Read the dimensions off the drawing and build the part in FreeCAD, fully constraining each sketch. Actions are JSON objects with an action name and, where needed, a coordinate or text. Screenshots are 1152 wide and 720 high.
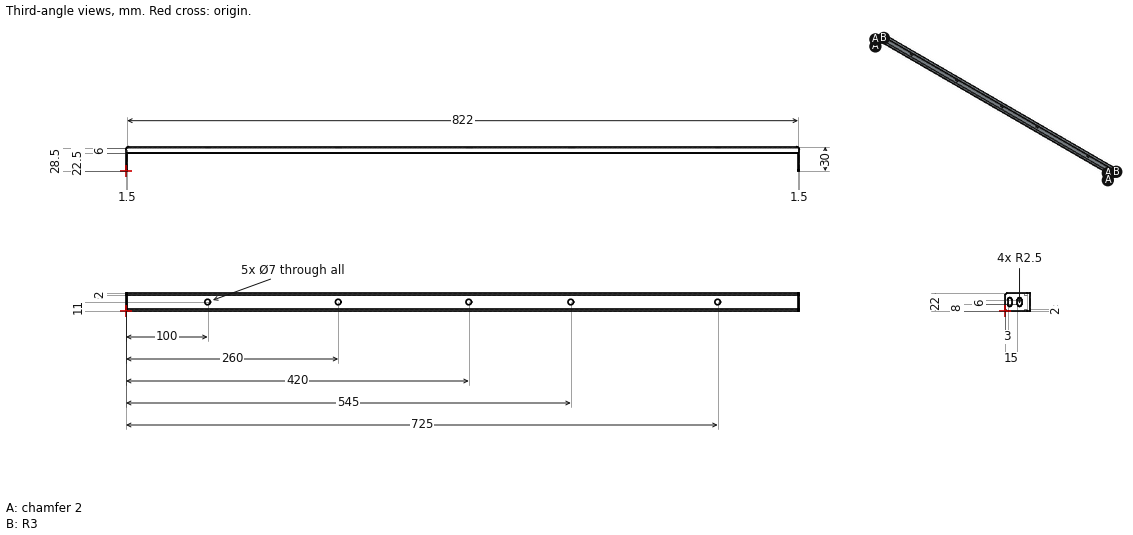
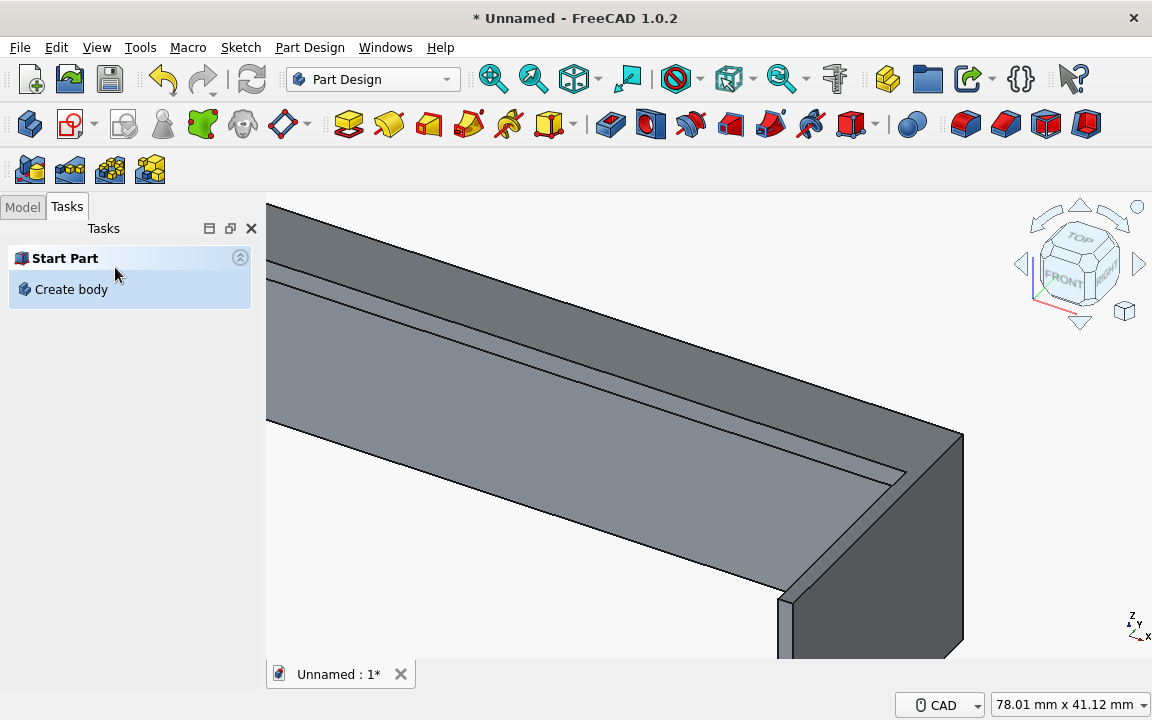
{"action": "left_click", "coordinate": [494, 80]}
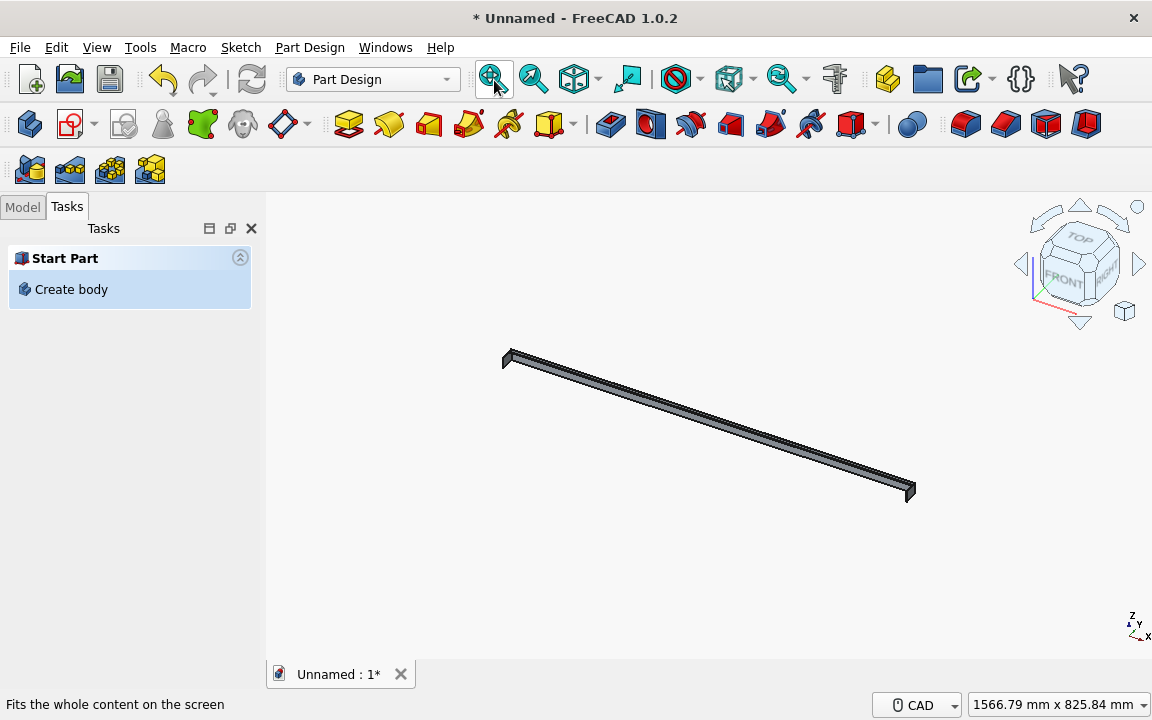
{"action": "key", "text": "5"}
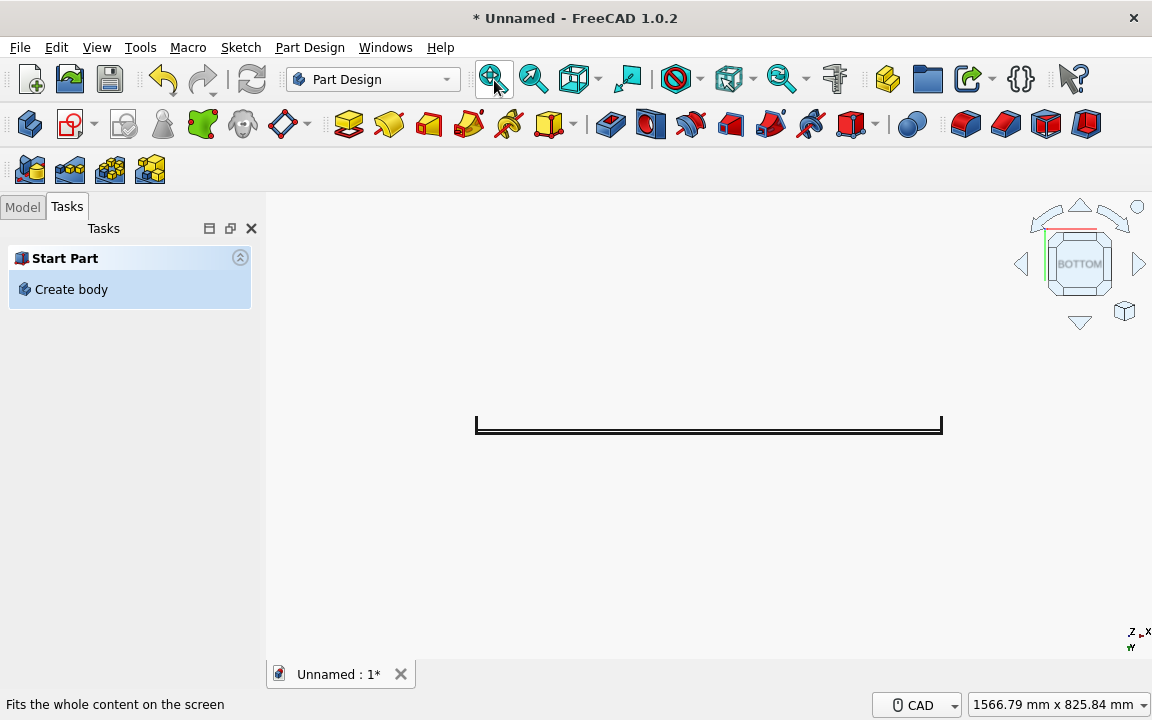
{"action": "scroll", "coordinate": [942, 427], "scroll_direction": "up", "scroll_amount": 15}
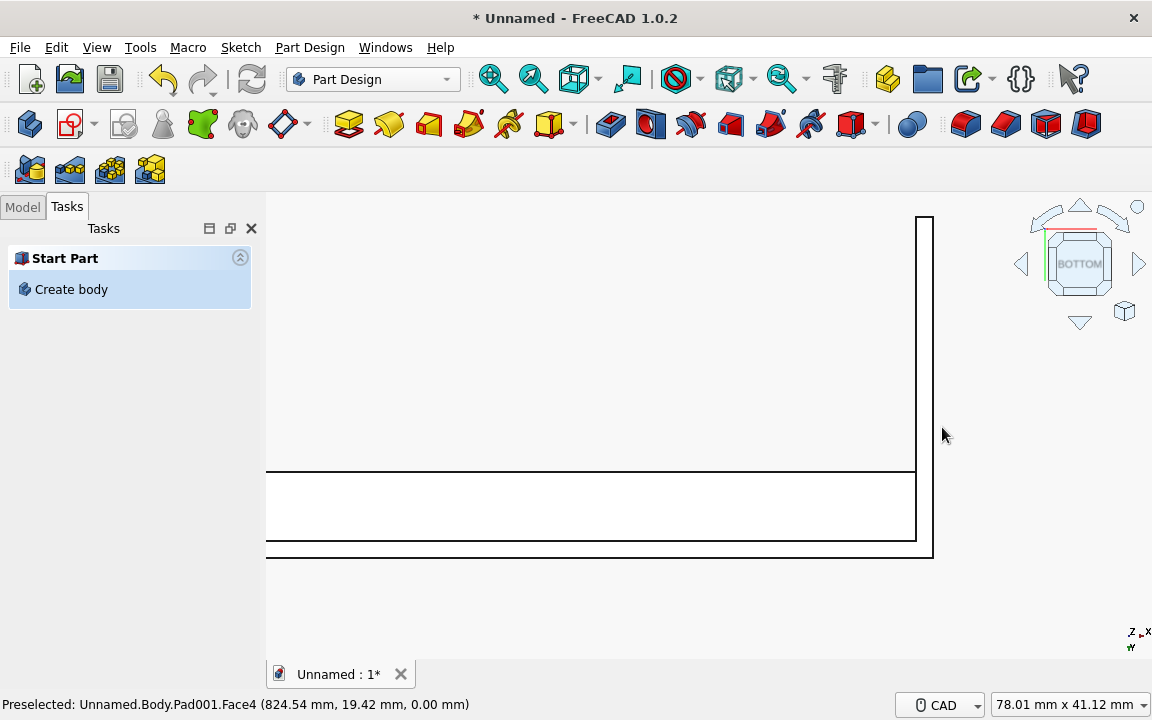
{"action": "scroll", "coordinate": [927, 437], "scroll_direction": "up", "scroll_amount": 4}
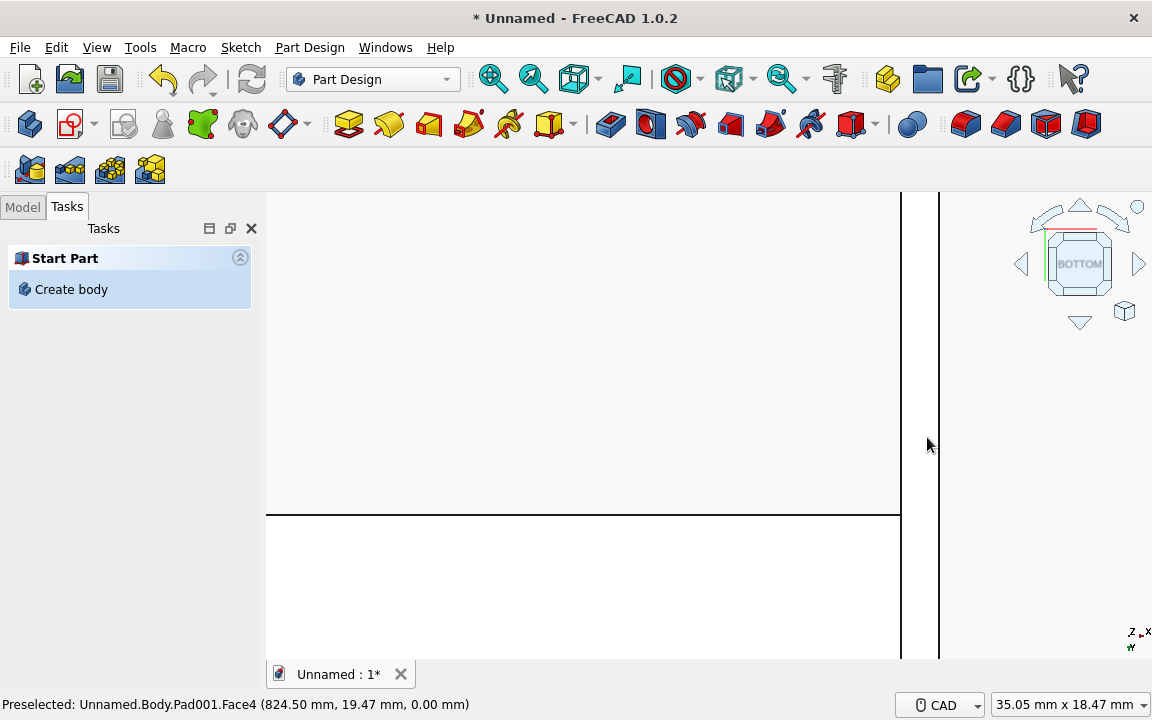
{"action": "left_click", "coordinate": [926, 438]}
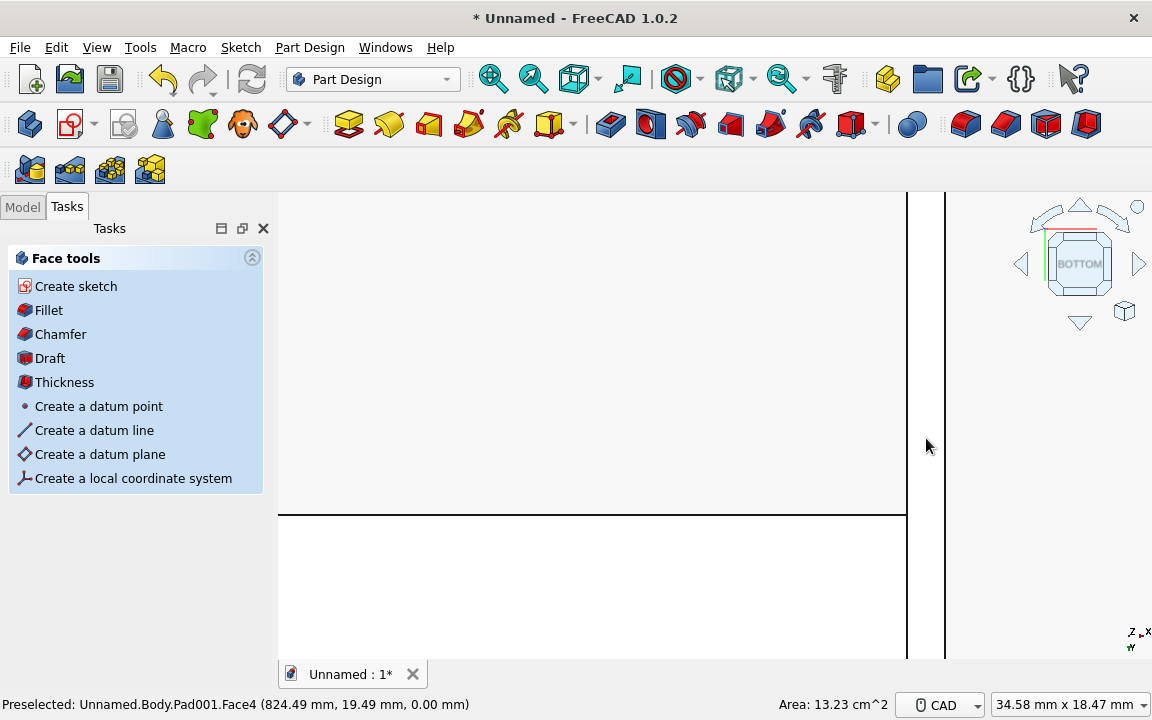
{"action": "left_click", "coordinate": [70, 124]}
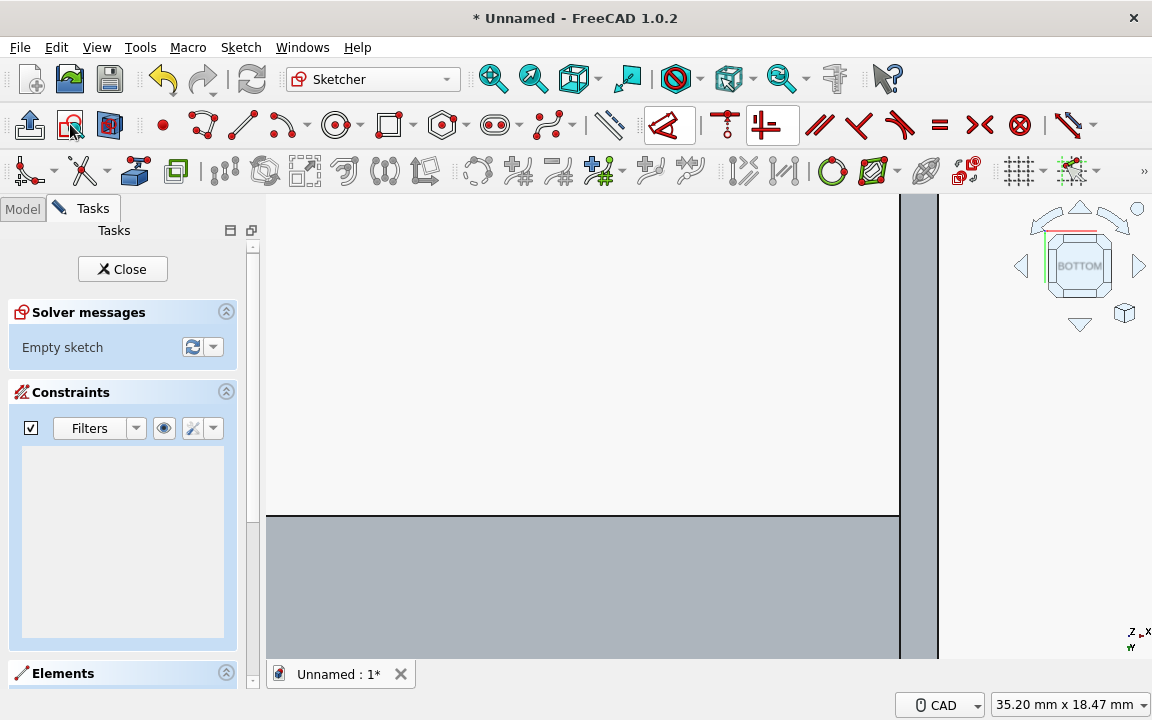
{"action": "scroll", "coordinate": [924, 430], "scroll_direction": "down", "scroll_amount": 18}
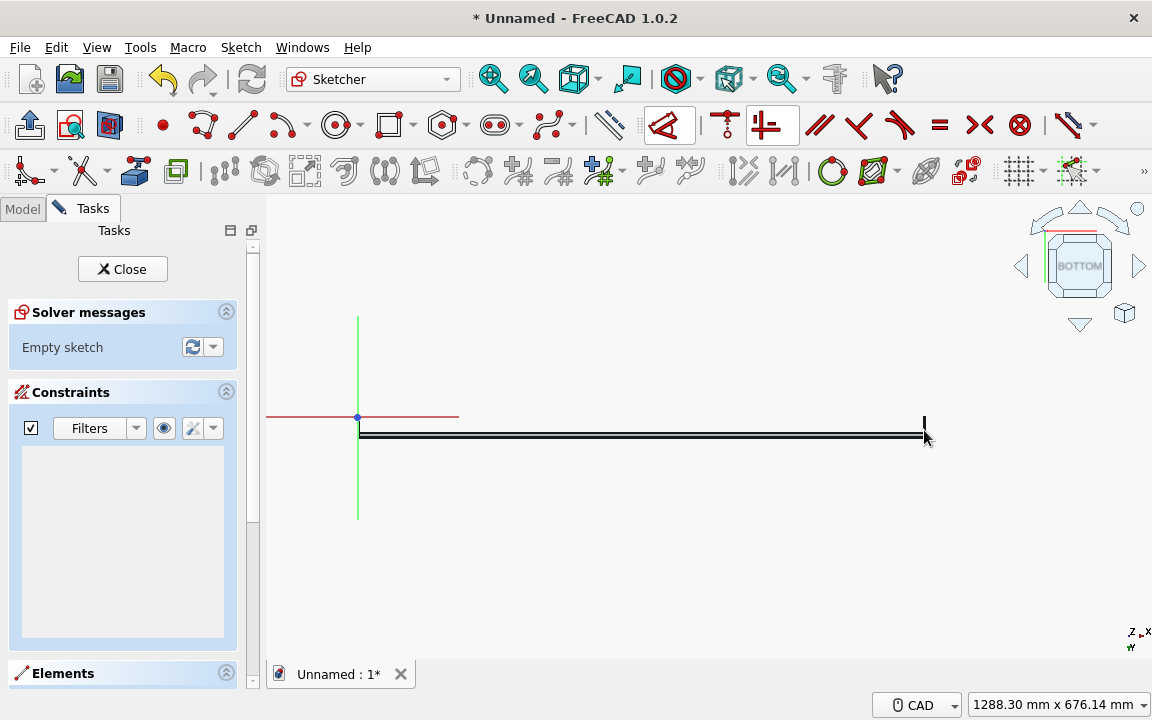
{"action": "left_click", "coordinate": [390, 126]}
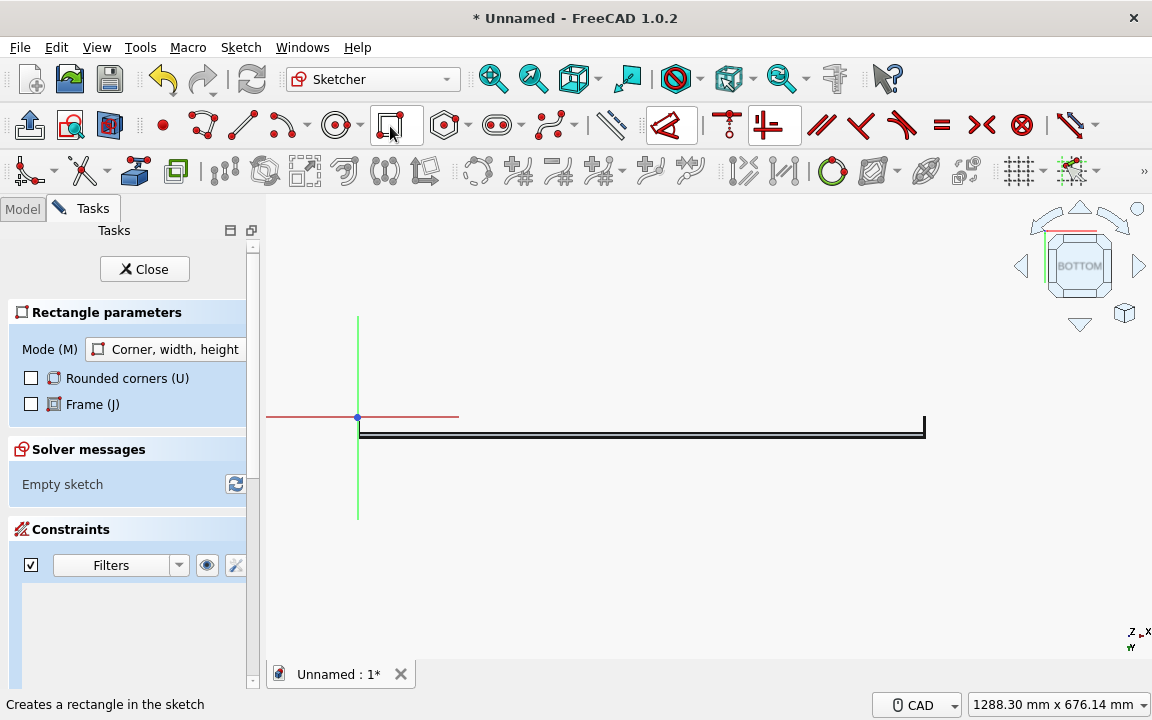
{"action": "scroll", "coordinate": [359, 433], "scroll_direction": "up", "scroll_amount": 14}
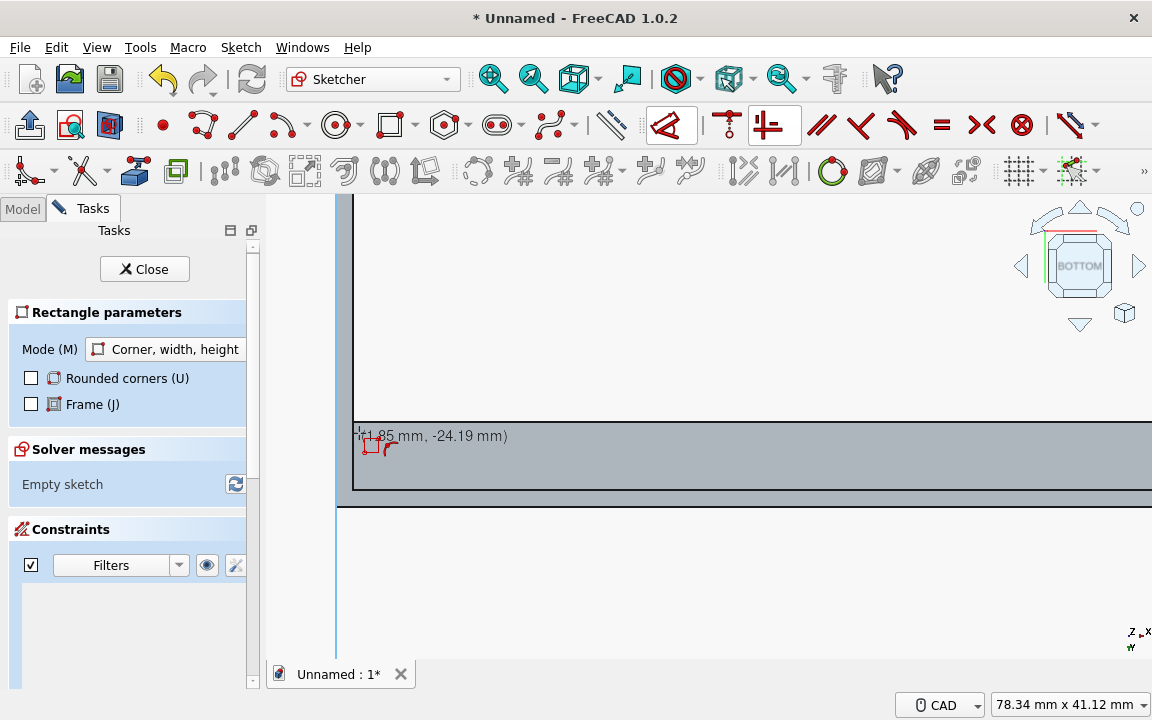
{"action": "left_click", "coordinate": [353, 422]}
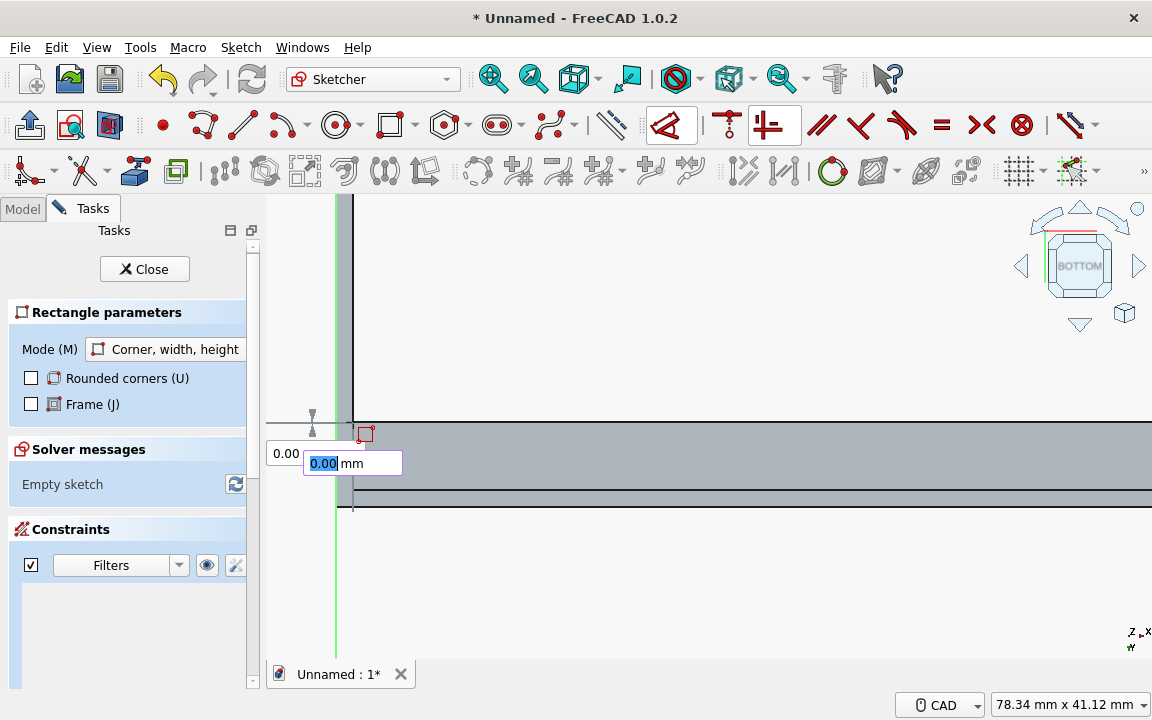
{"action": "scroll", "coordinate": [412, 432], "scroll_direction": "down", "scroll_amount": 15}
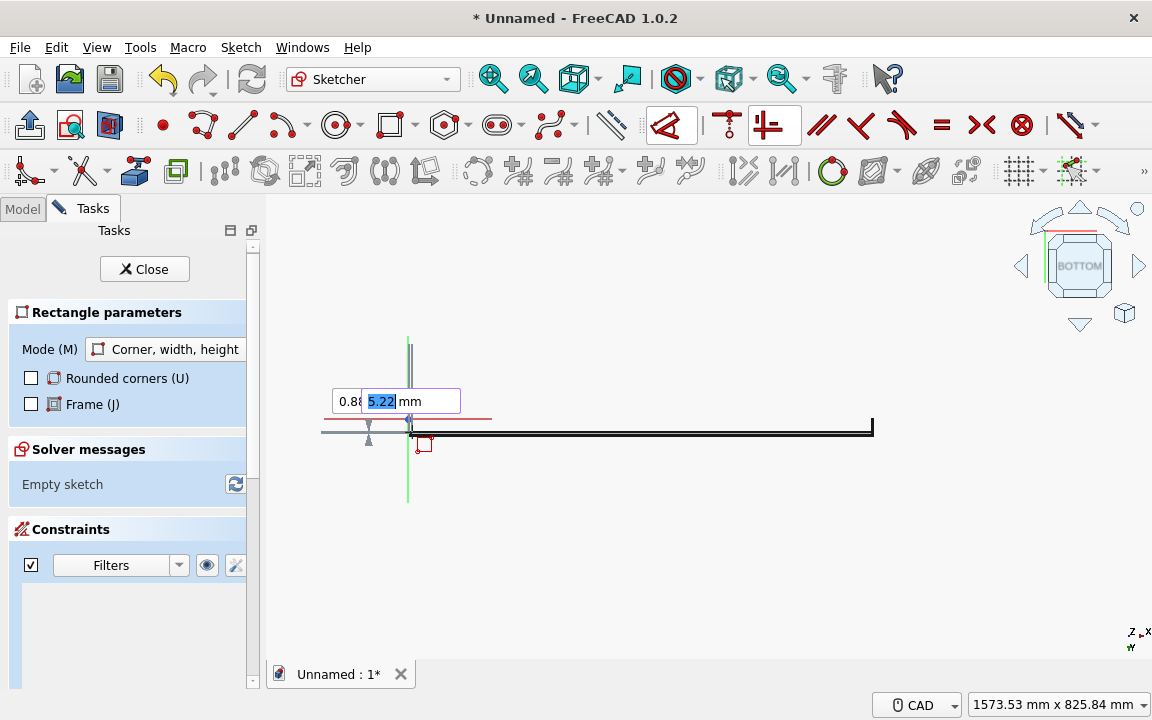
{"action": "left_click", "coordinate": [872, 435]}
{"action": "key", "text": "Escape"}